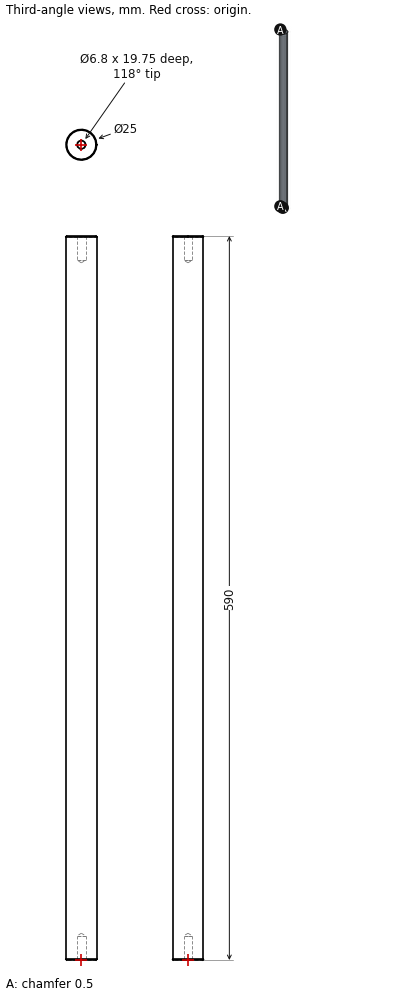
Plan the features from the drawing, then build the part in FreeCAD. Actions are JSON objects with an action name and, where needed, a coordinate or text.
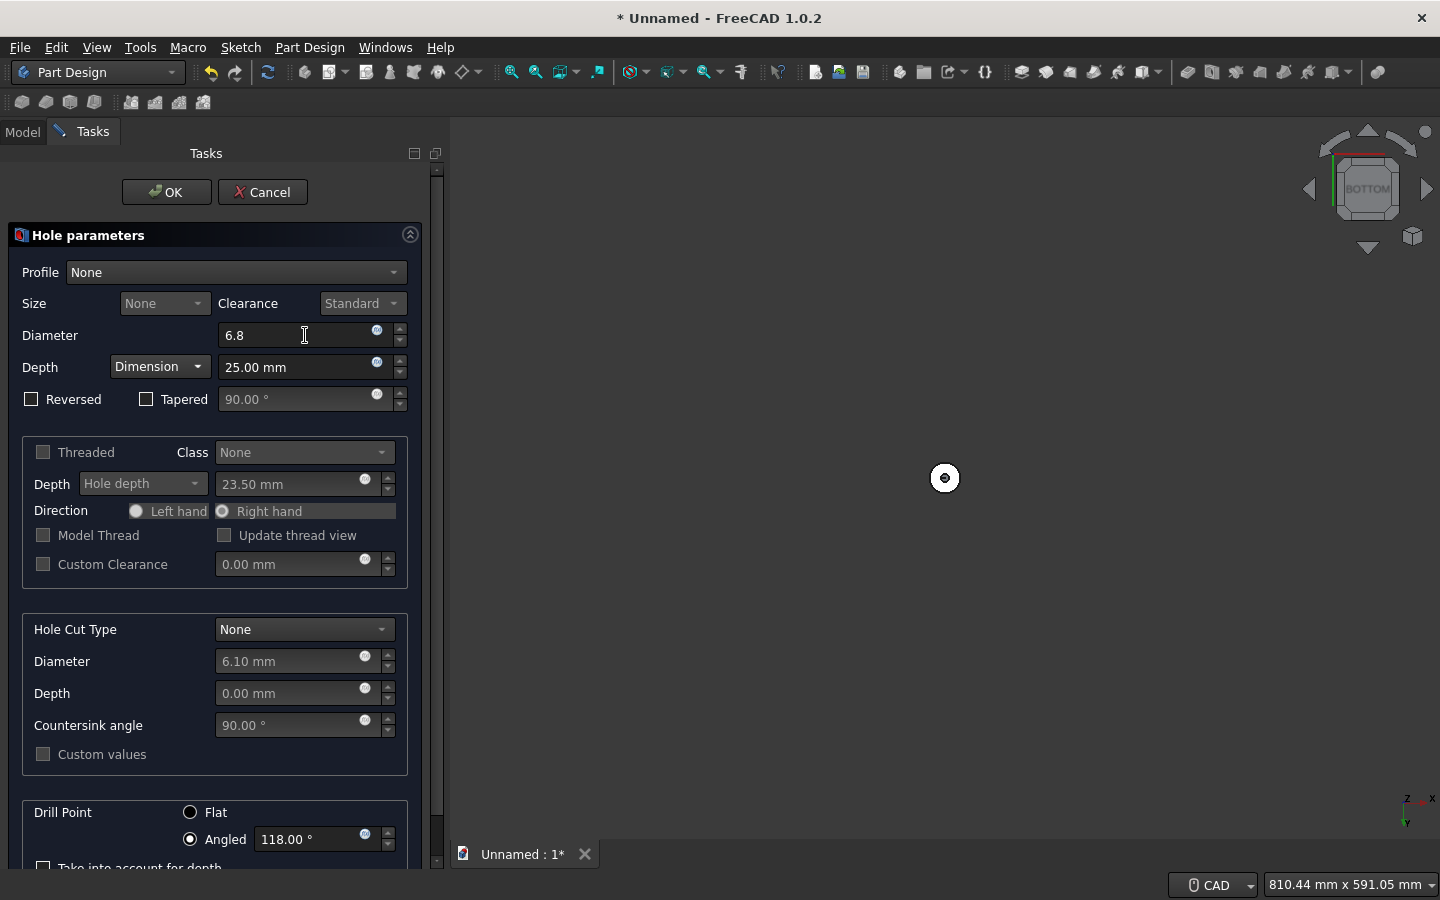
{"action": "triple_click", "coordinate": [305, 367]}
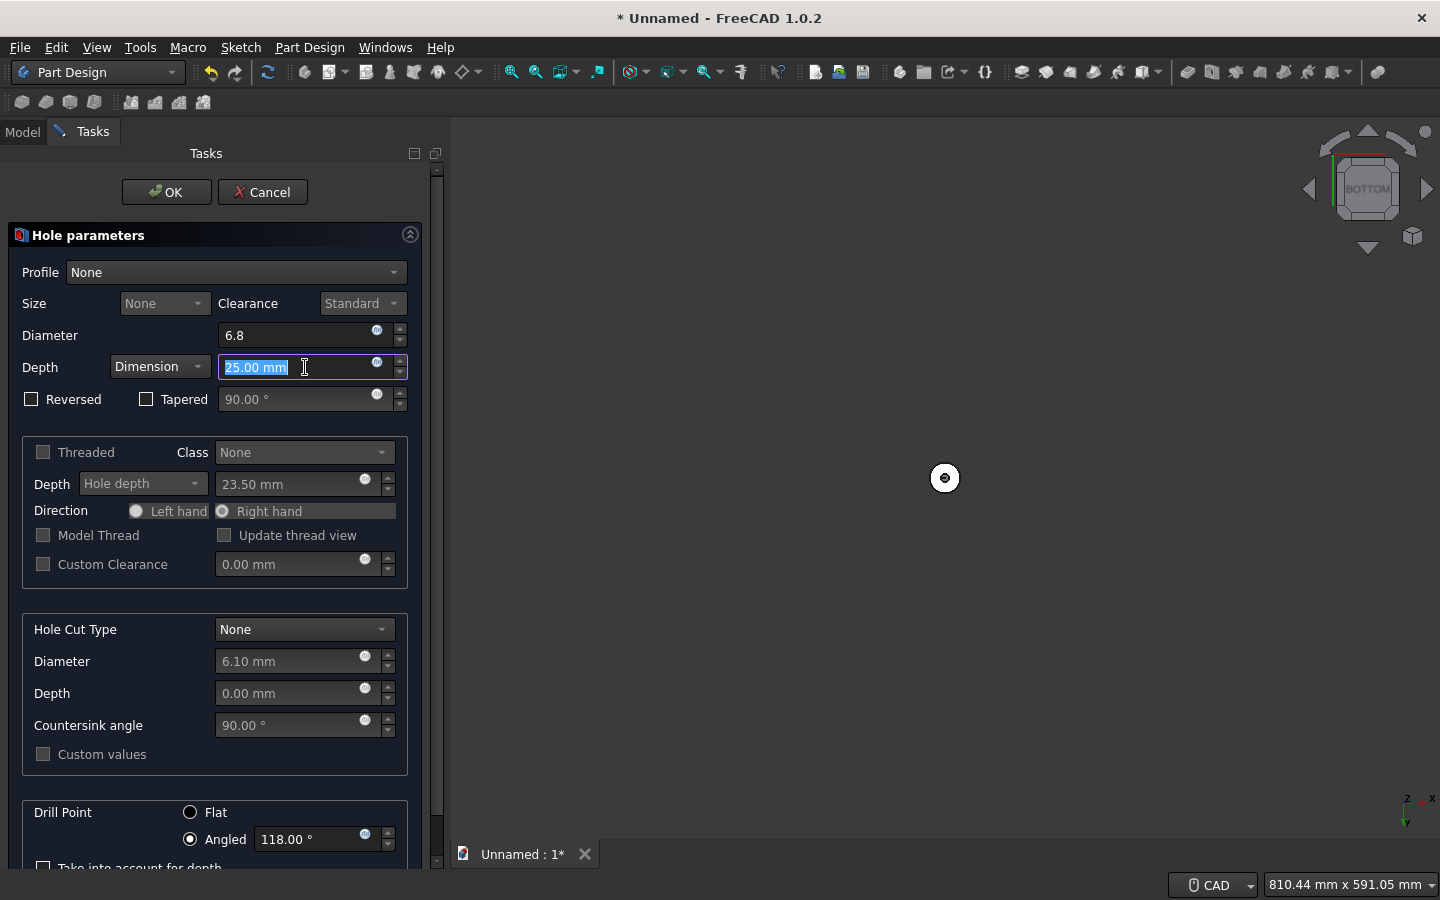
{"action": "type", "text": "19.75"}
{"action": "key", "text": "Tab"}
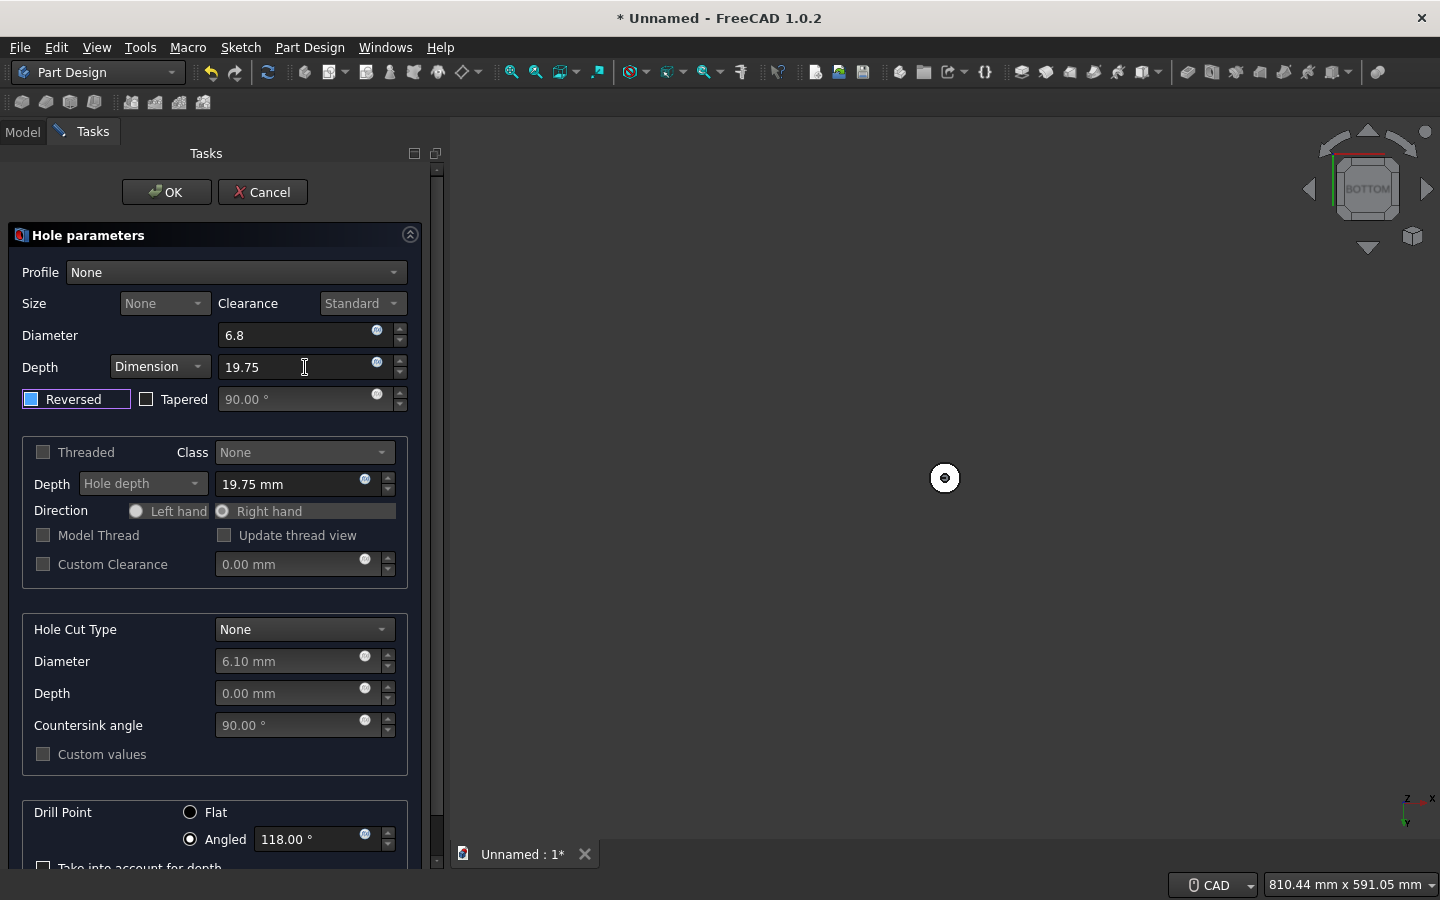
{"action": "left_click", "coordinate": [167, 192]}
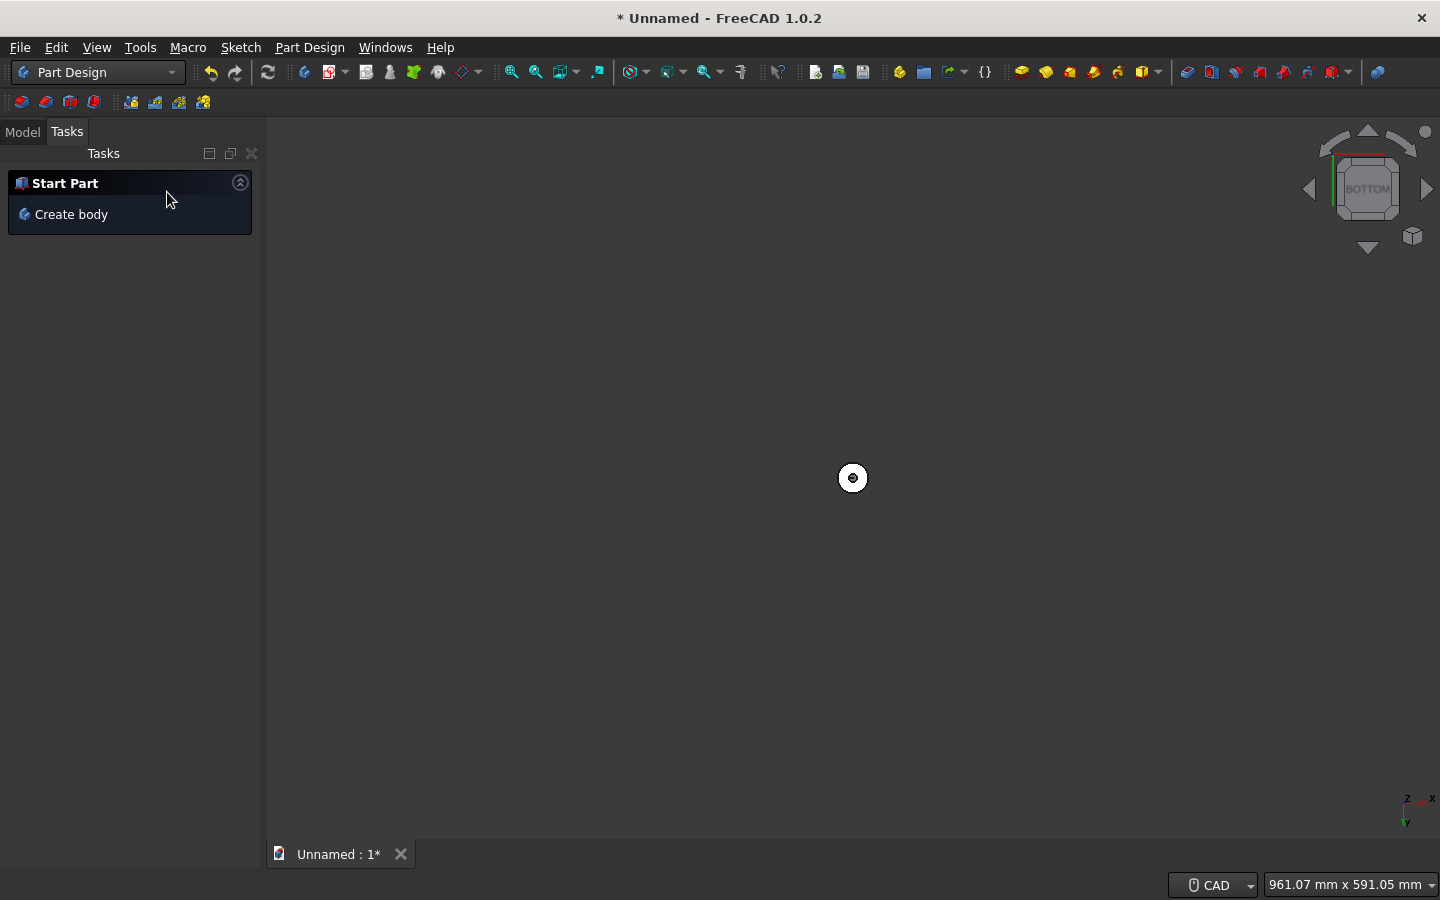
{"action": "key", "text": "v f"}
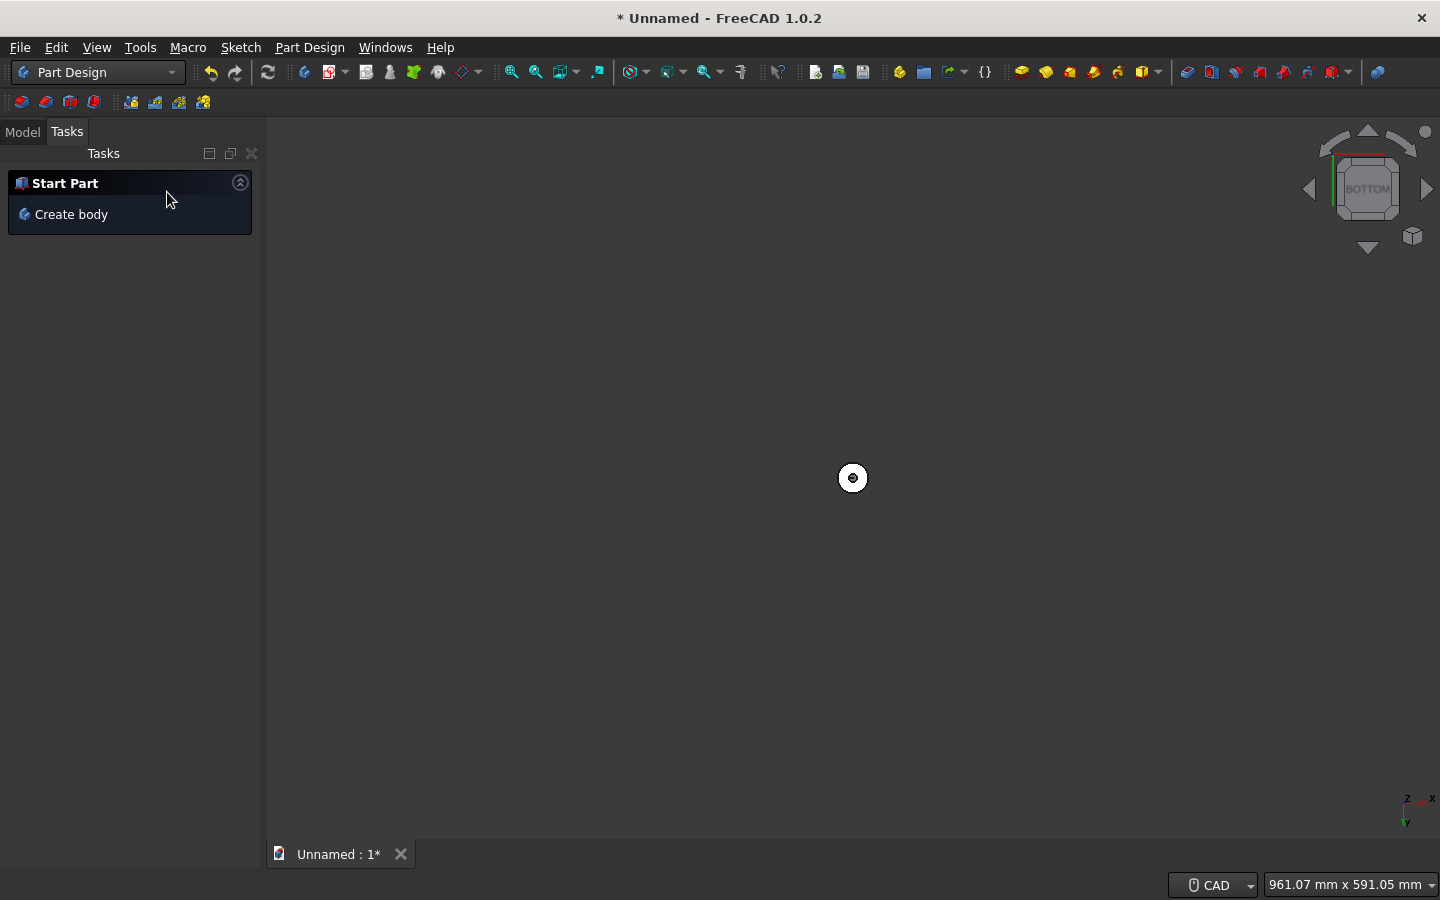
{"action": "left_click", "coordinate": [857, 477]}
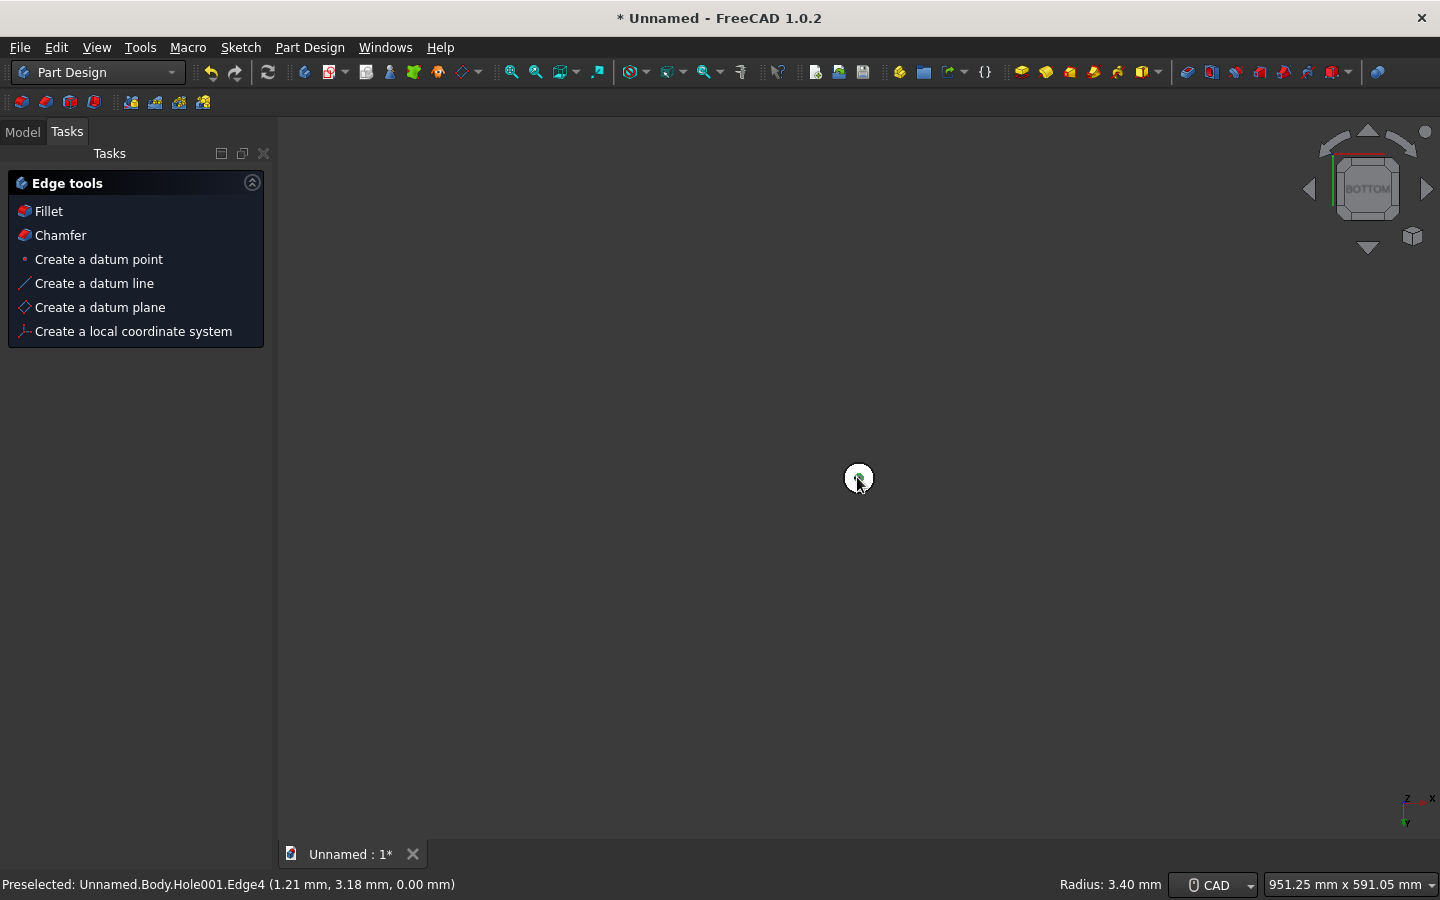
{"action": "left_click", "coordinate": [844, 477], "text": "ctrl"}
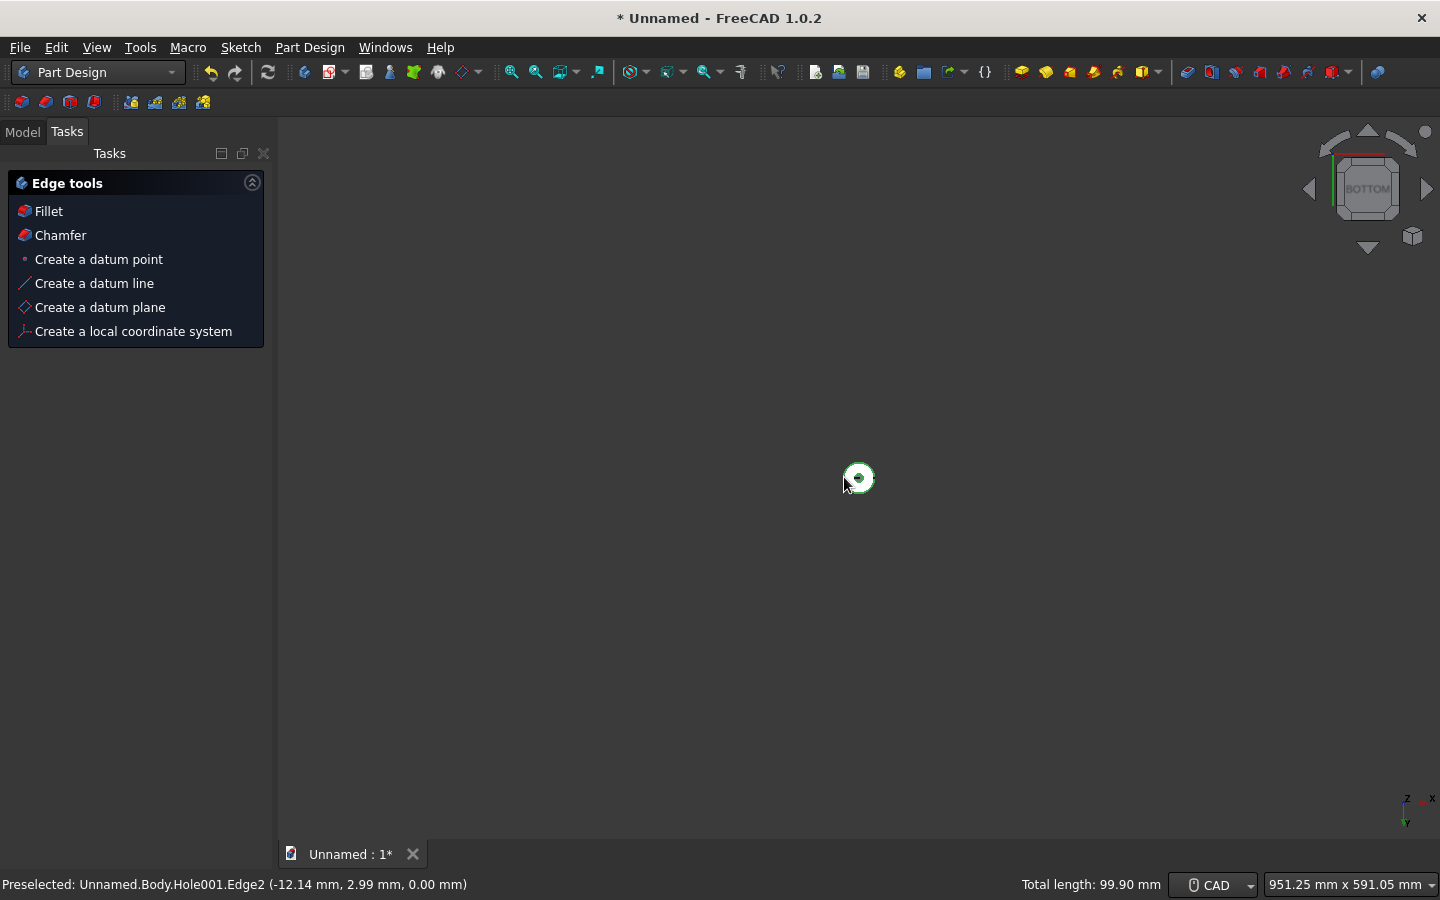
{"action": "key", "text": "0"}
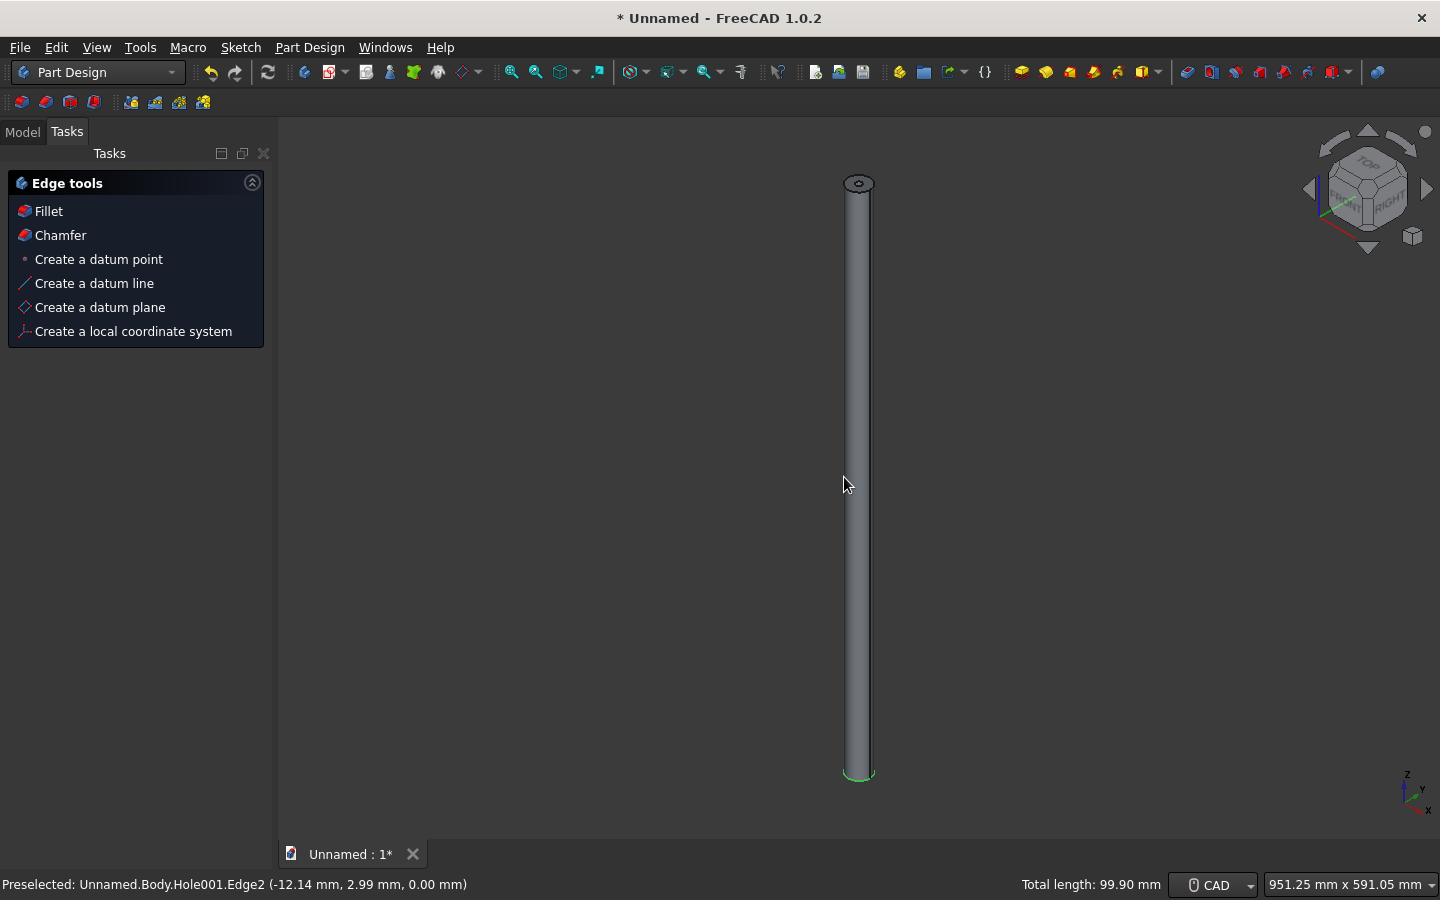
{"action": "left_click", "coordinate": [848, 177], "text": "ctrl"}